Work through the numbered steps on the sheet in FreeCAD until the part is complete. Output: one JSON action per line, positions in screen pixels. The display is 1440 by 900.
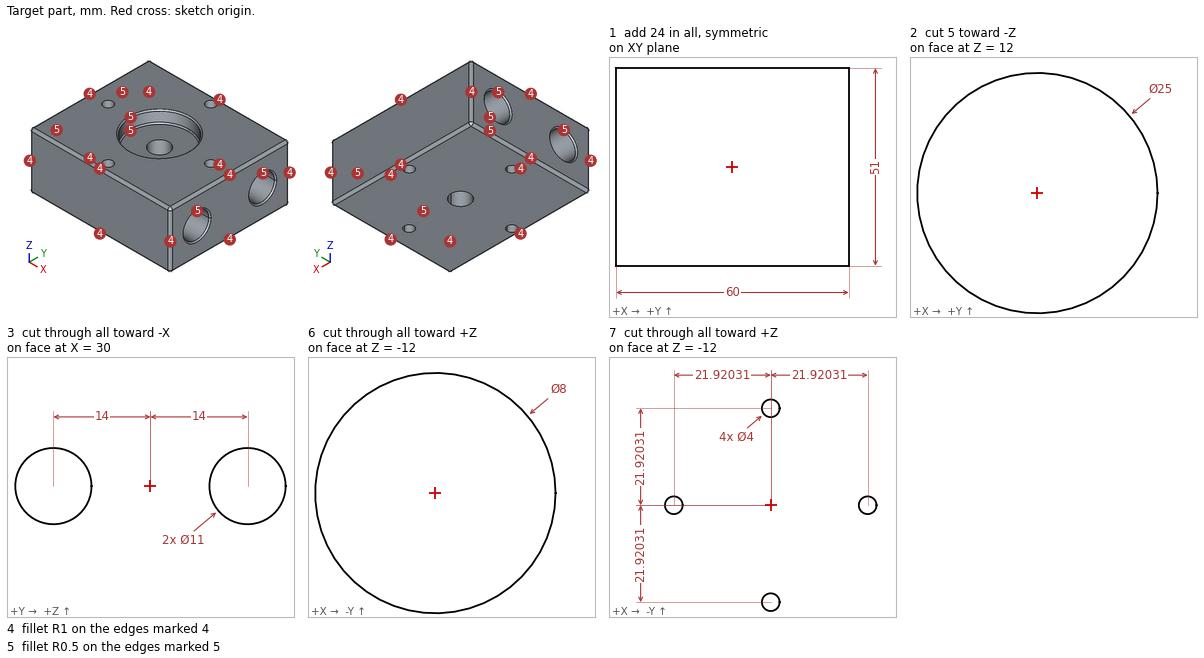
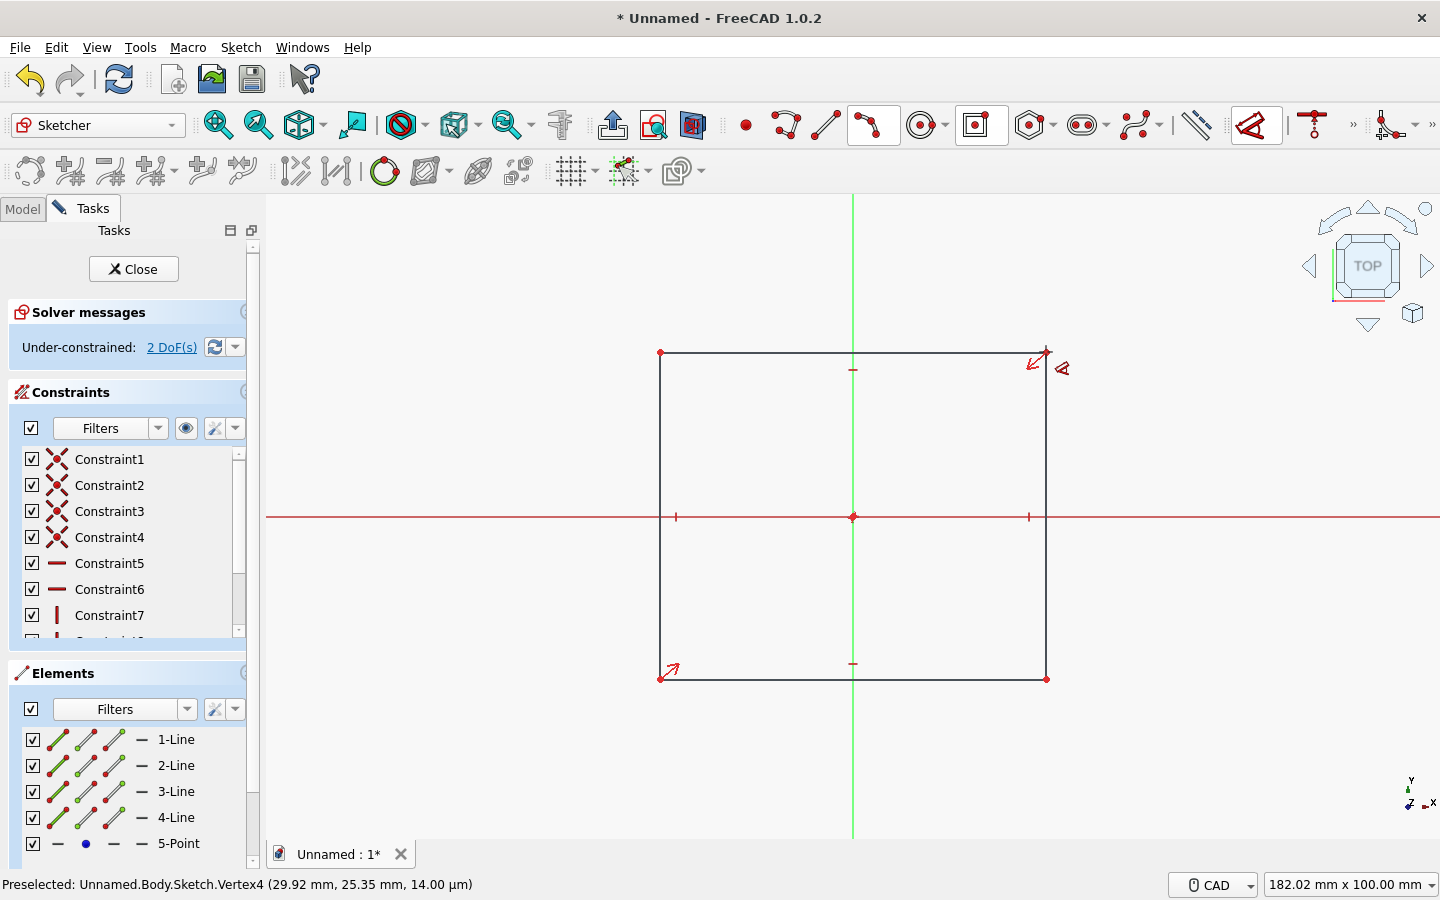
{"action": "left_click", "coordinate": [776, 680]}
{"action": "left_click", "coordinate": [764, 714]}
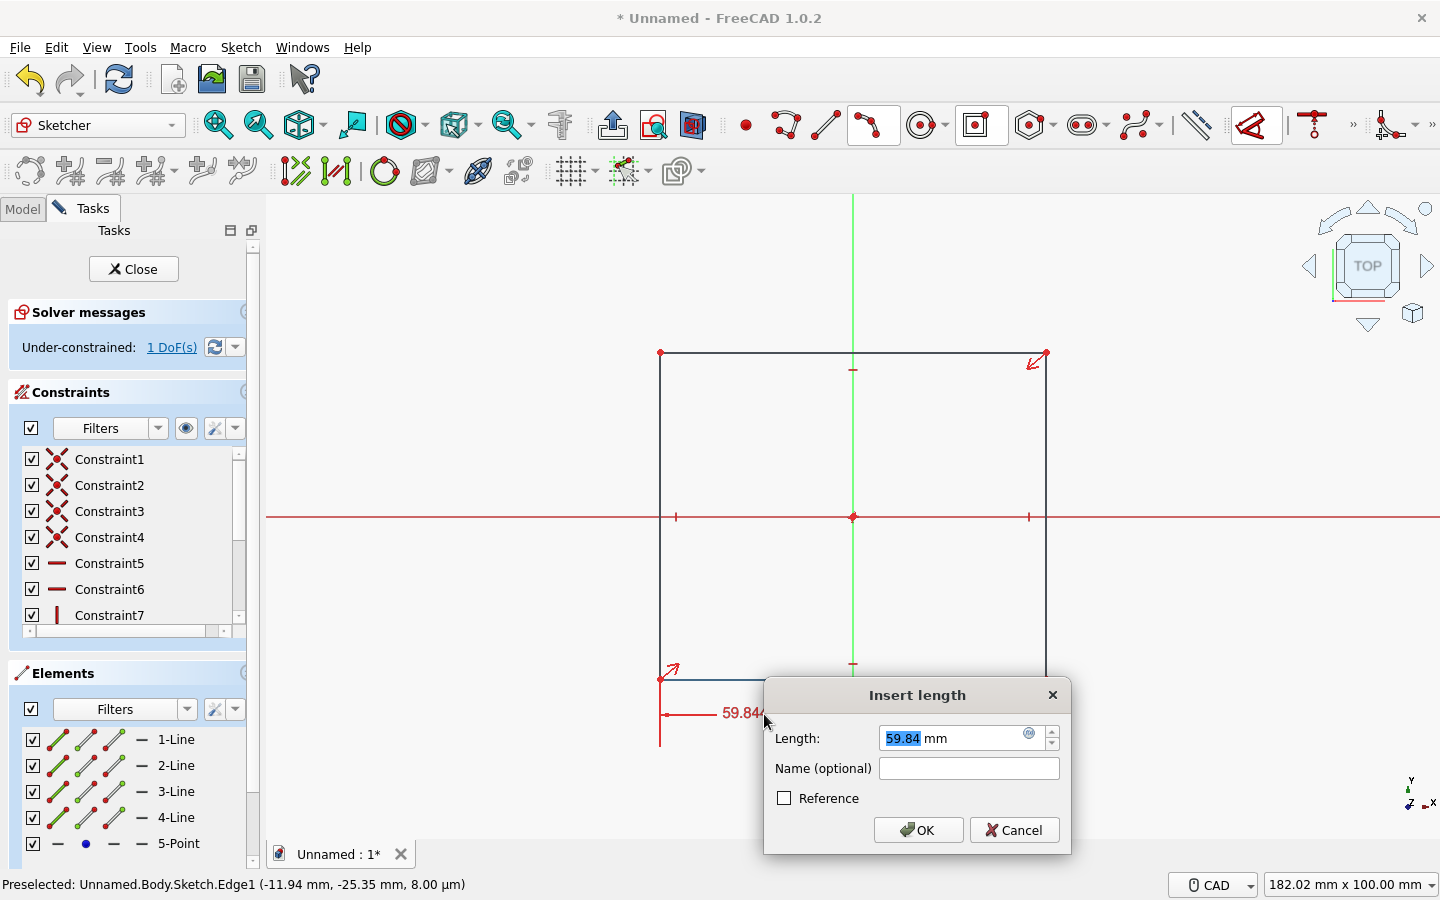
{"action": "type", "text": "60"}
{"action": "key", "text": "Return"}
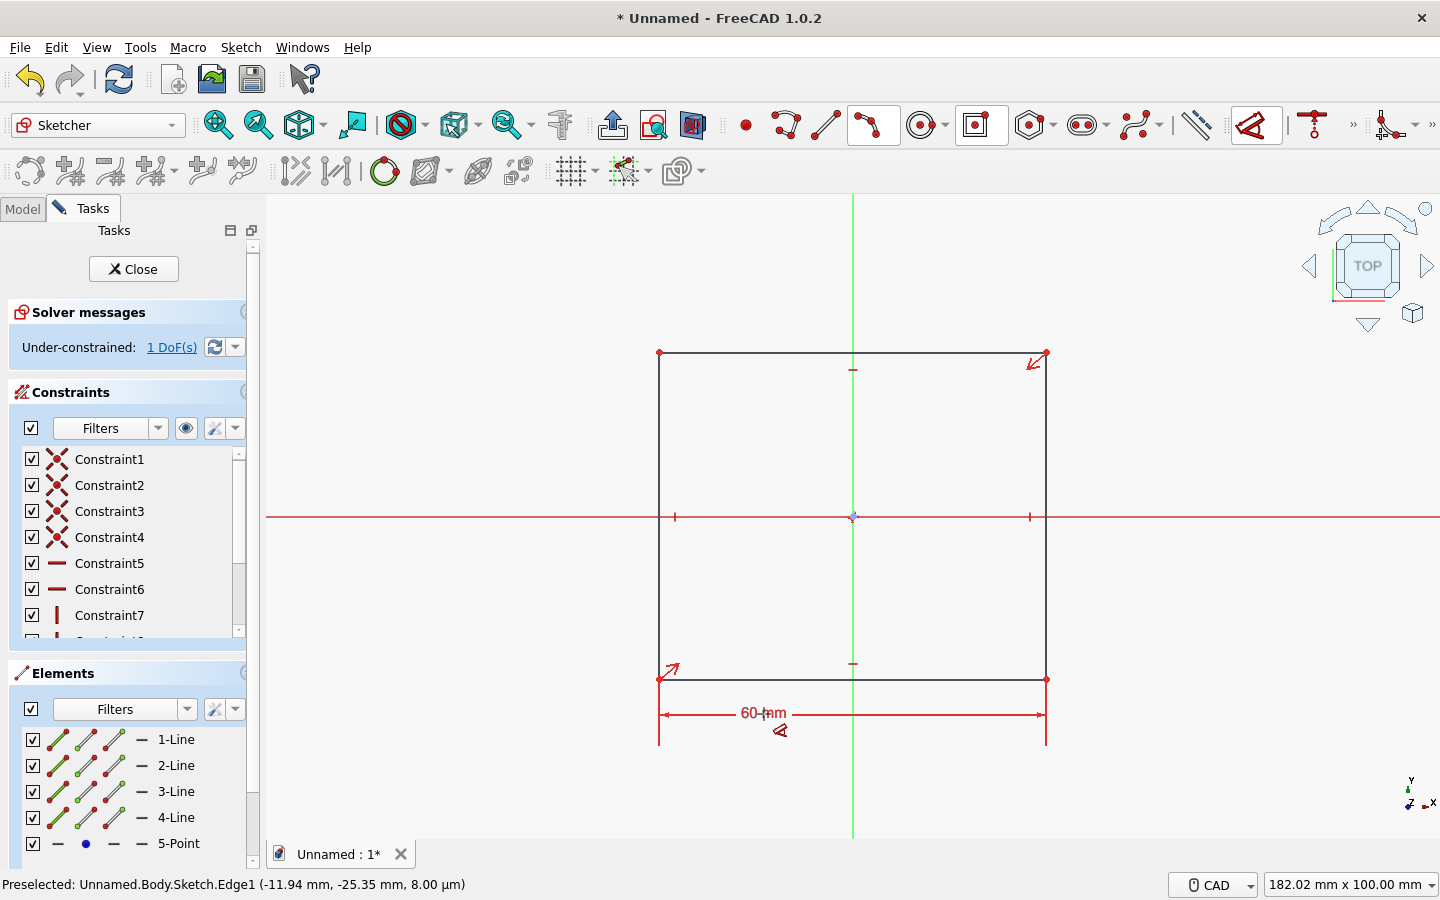
{"action": "left_click", "coordinate": [1046, 582]}
{"action": "left_click", "coordinate": [1080, 441]}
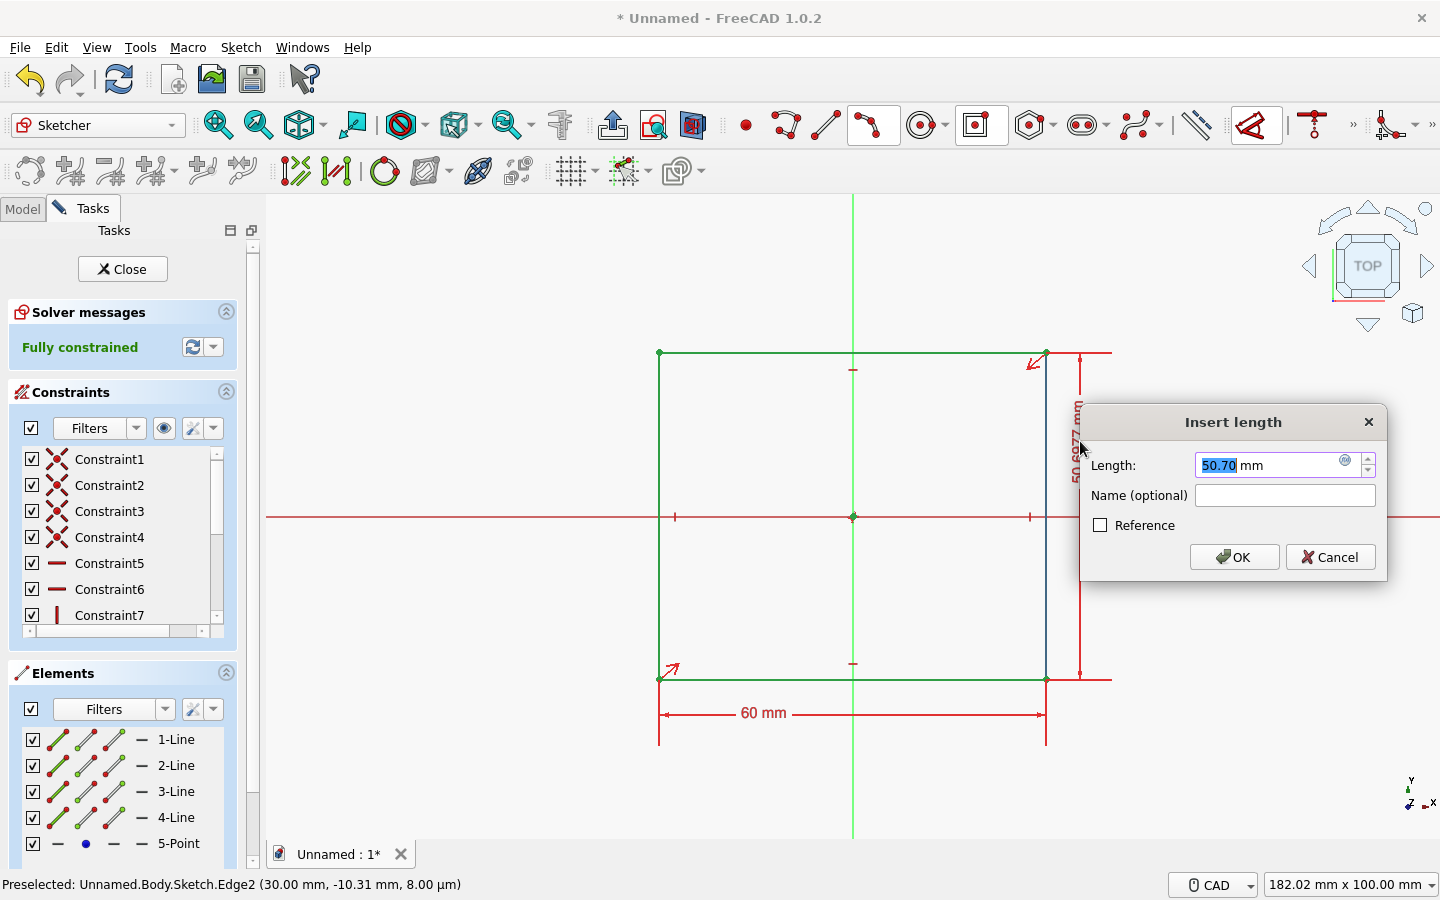
{"action": "type", "text": "51"}
{"action": "key", "text": "Return"}
{"action": "key", "text": "Escape"}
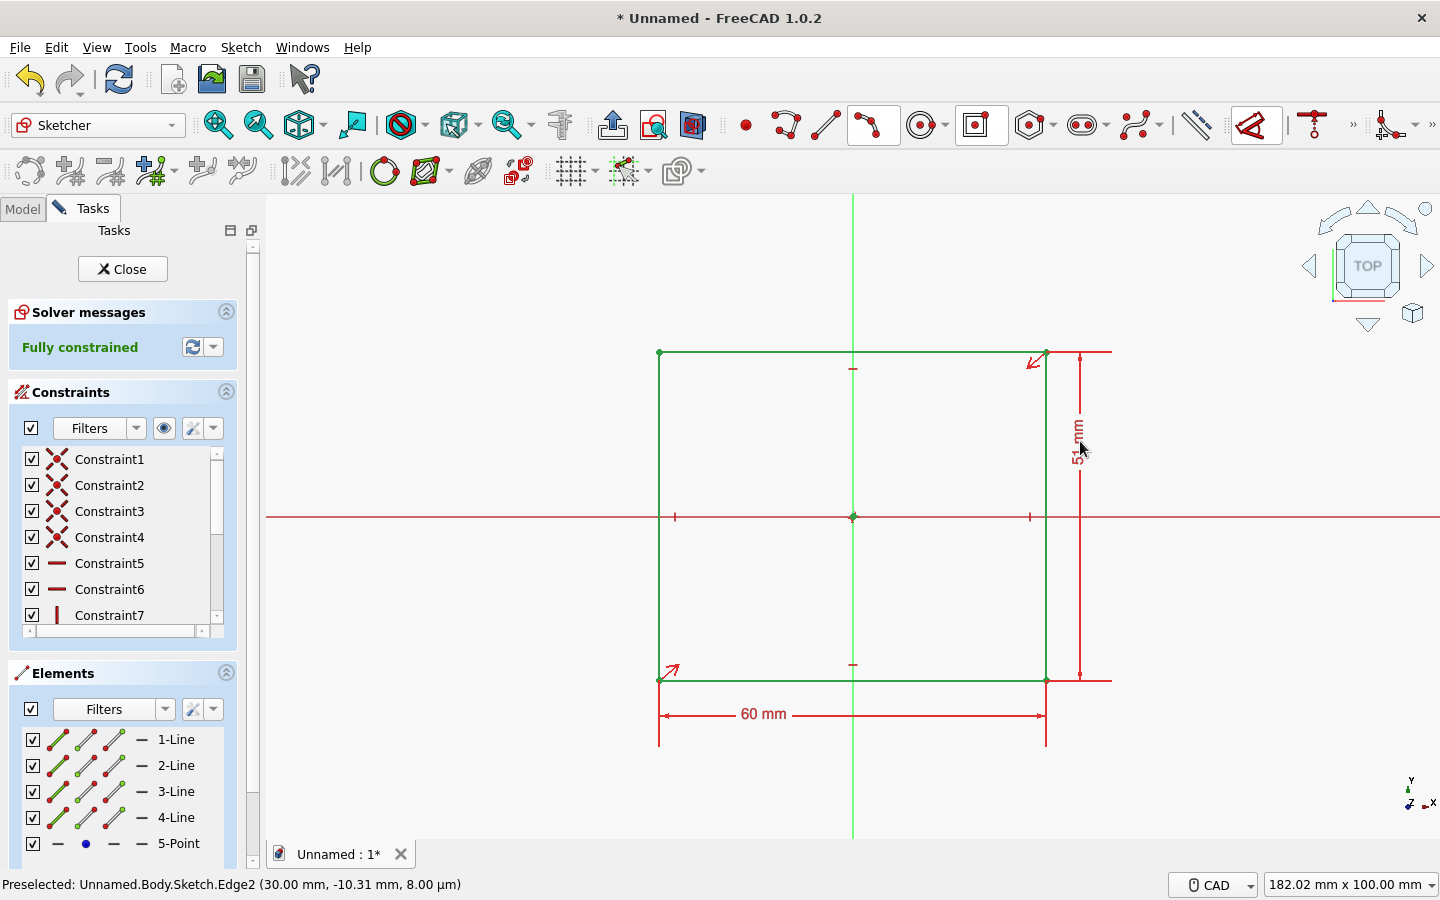
{"action": "left_click", "coordinate": [123, 269]}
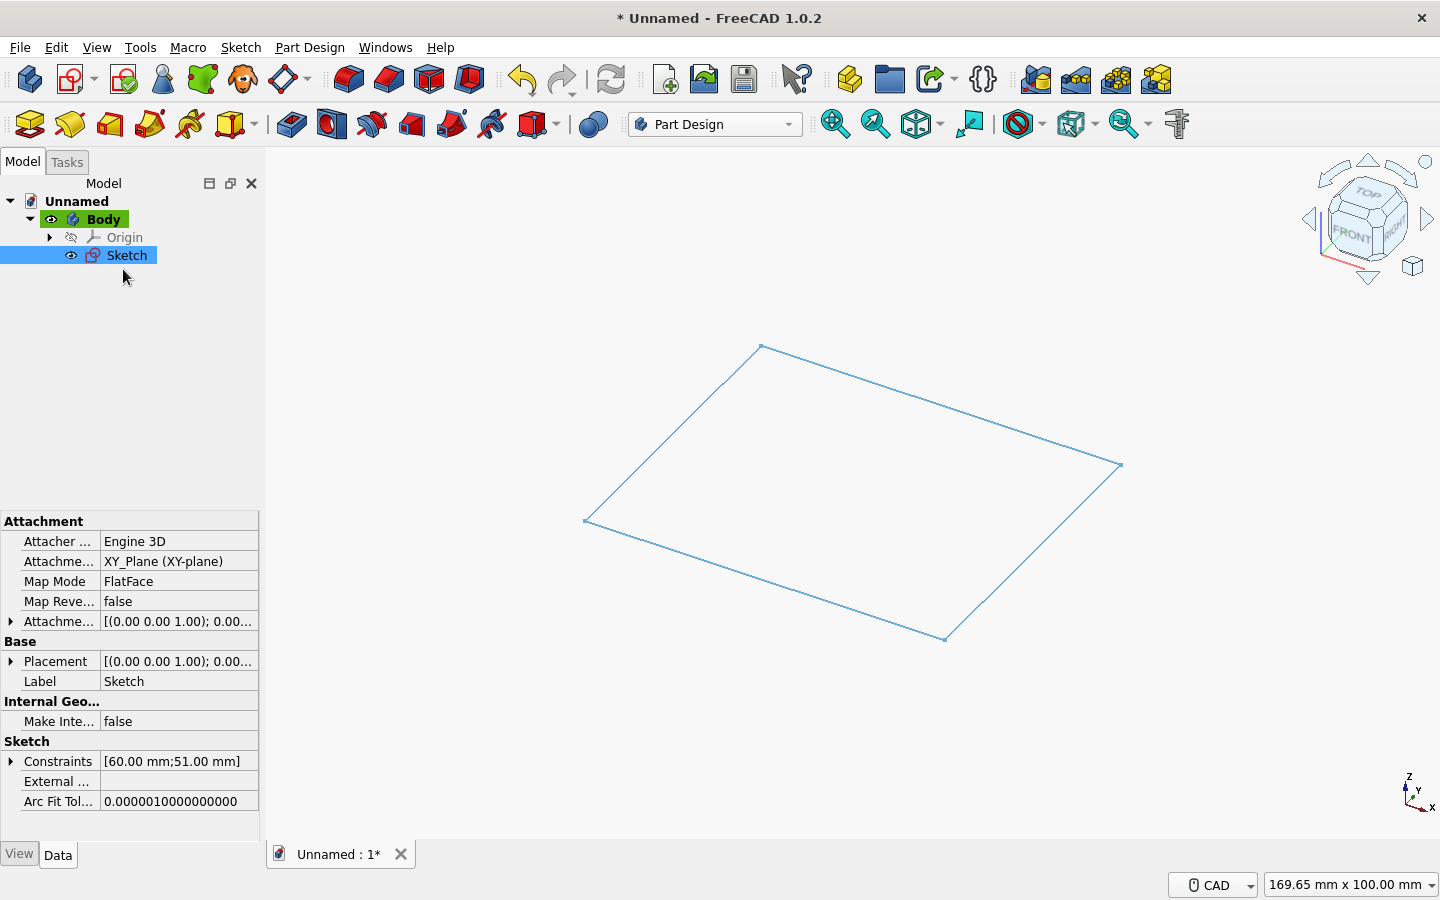
{"action": "left_click", "coordinate": [30, 124]}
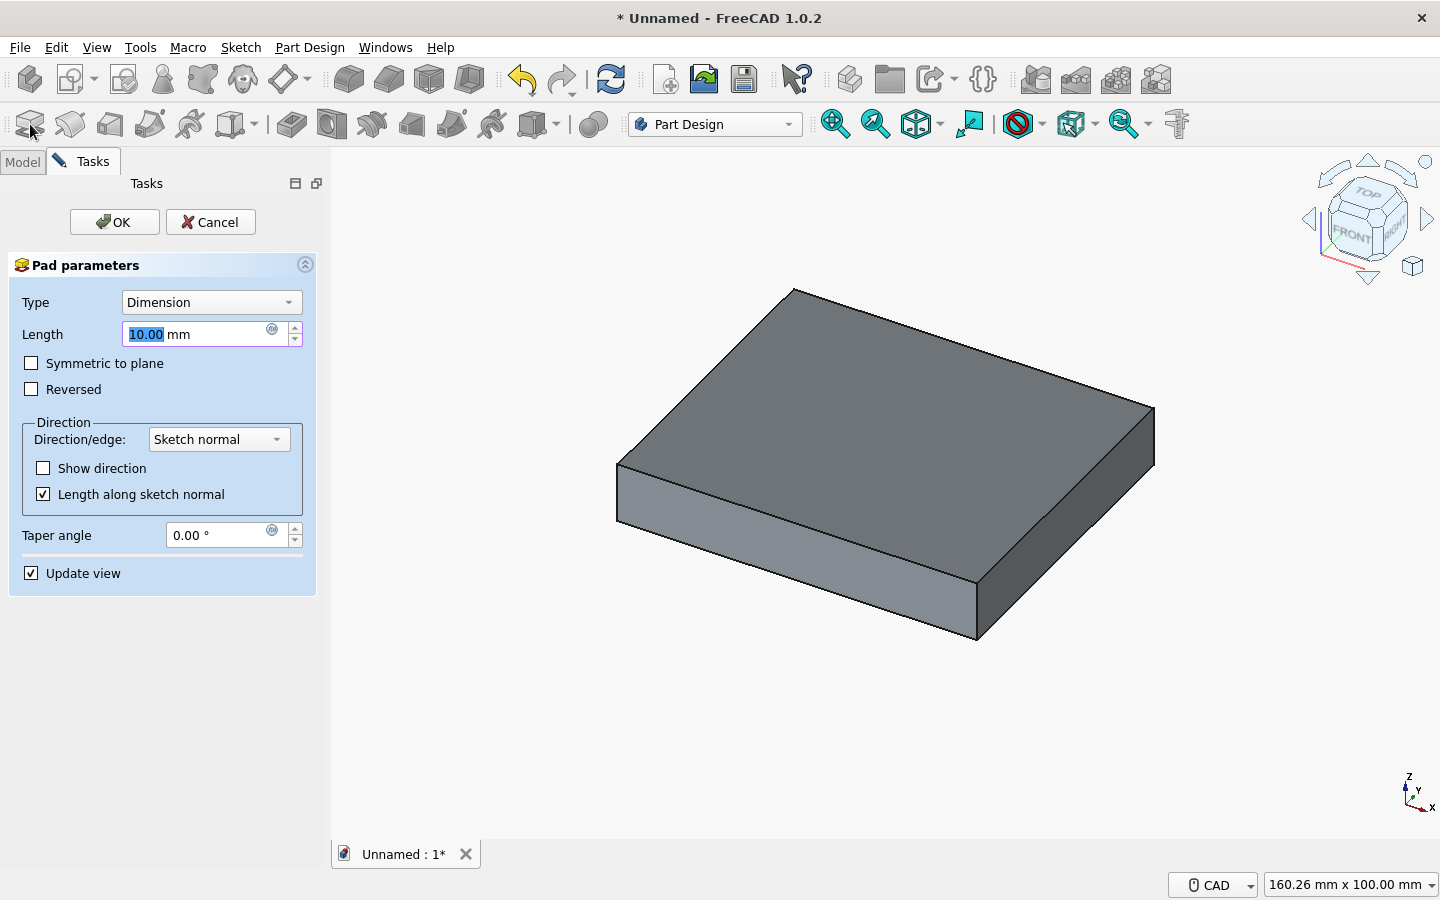
{"action": "type", "text": "24"}
{"action": "key", "text": "Tab"}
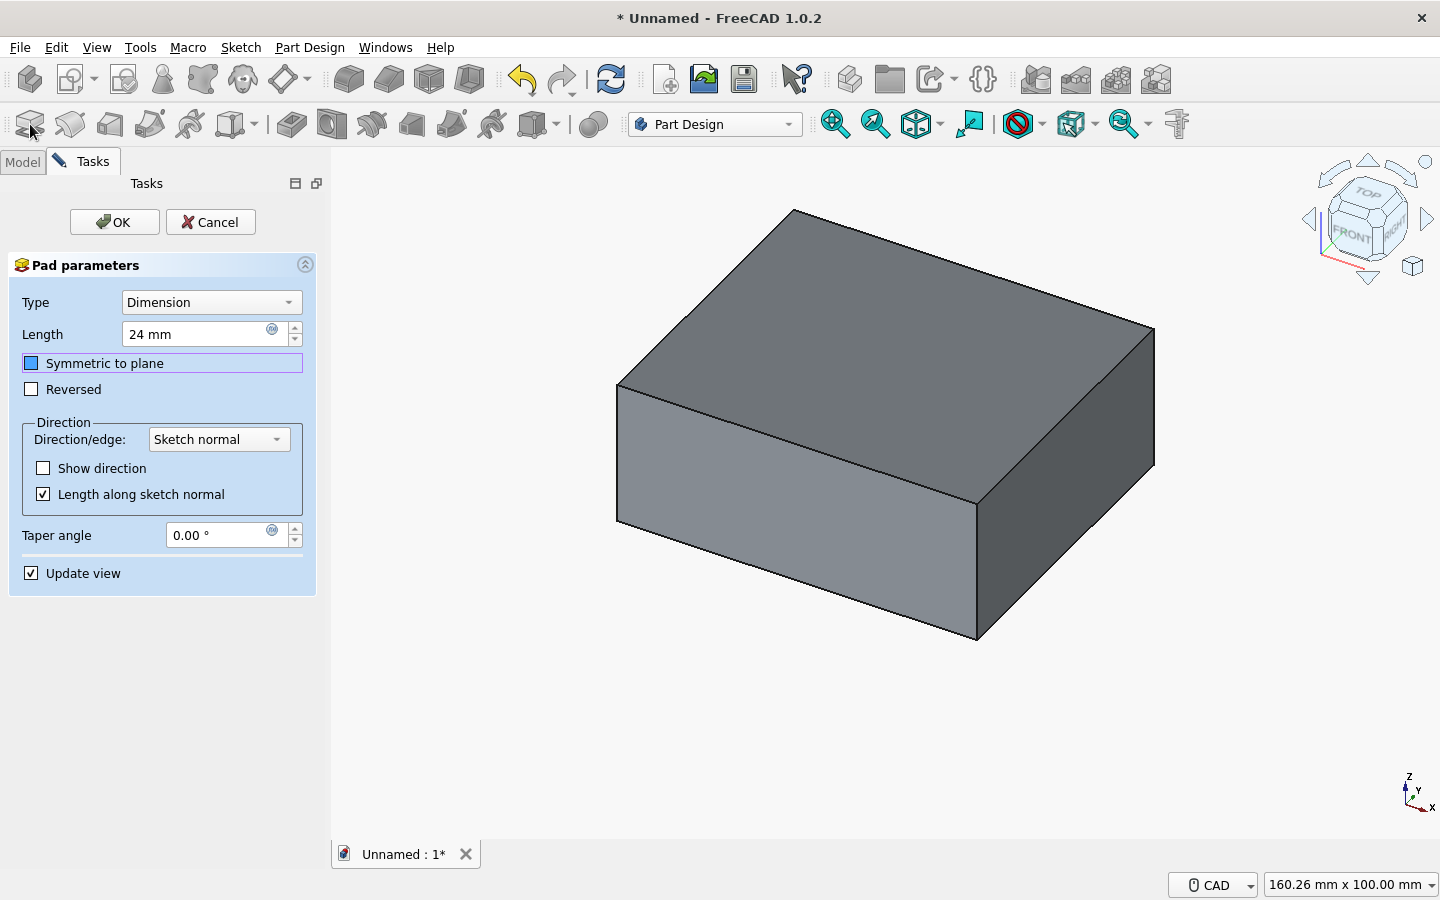
{"action": "left_click", "coordinate": [30, 363]}